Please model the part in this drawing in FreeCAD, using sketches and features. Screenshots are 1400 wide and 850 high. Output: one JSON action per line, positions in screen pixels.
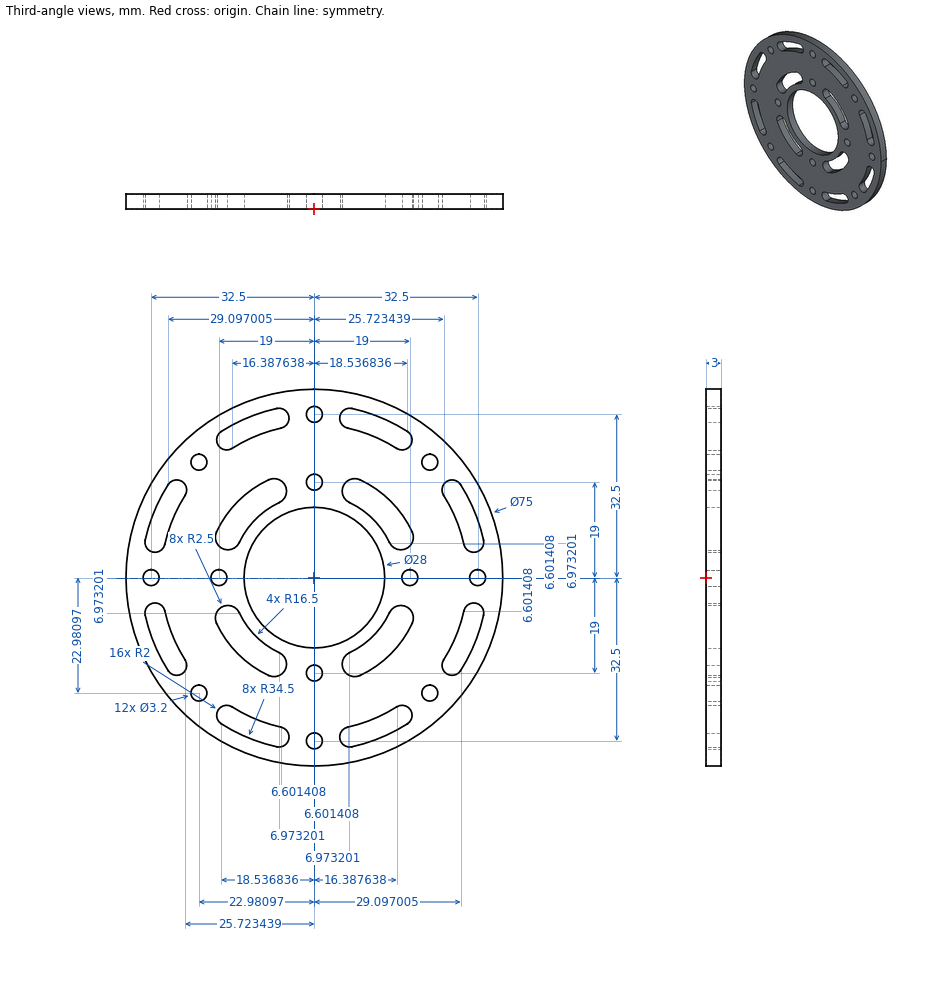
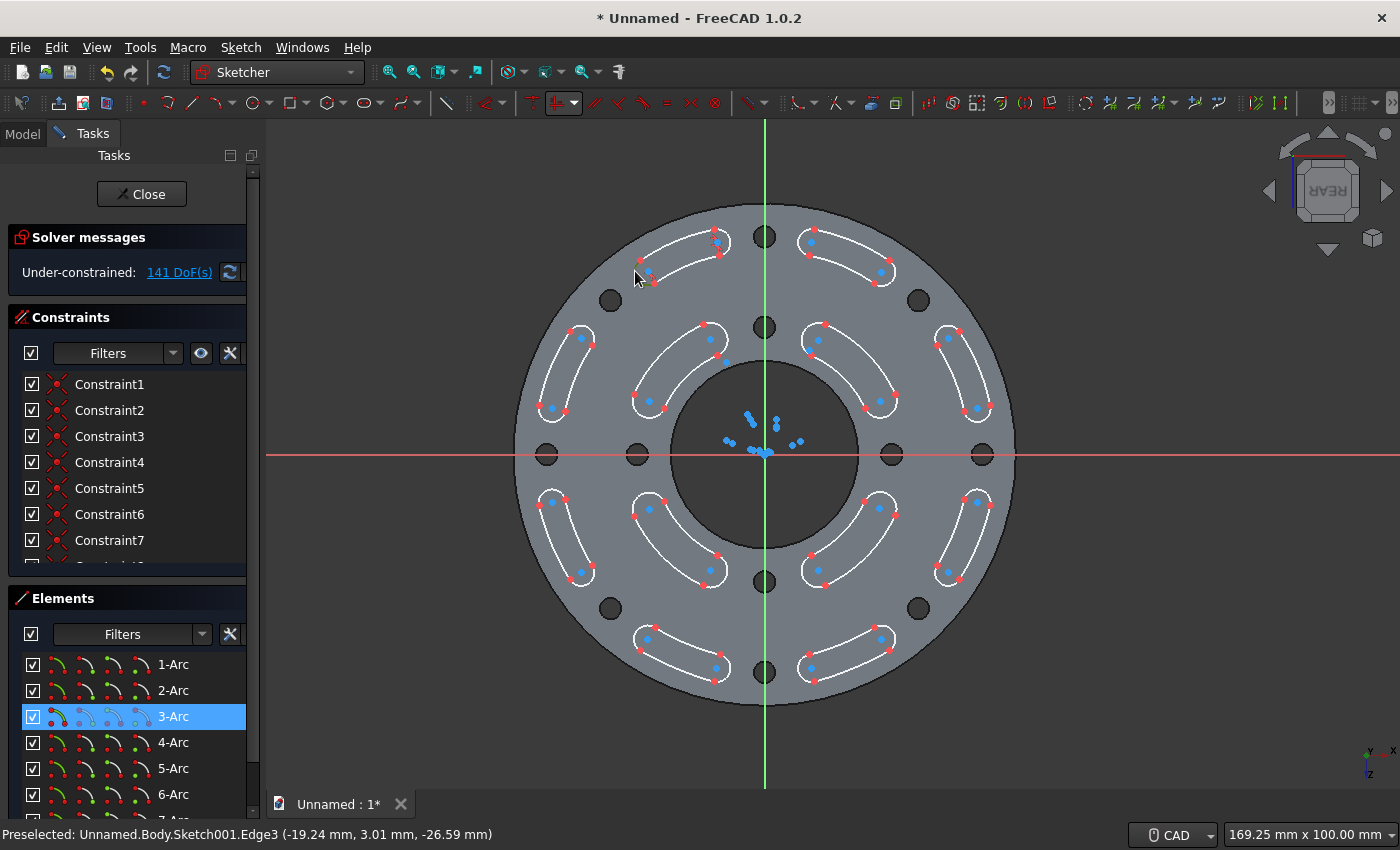
{"action": "left_click", "coordinate": [699, 261]}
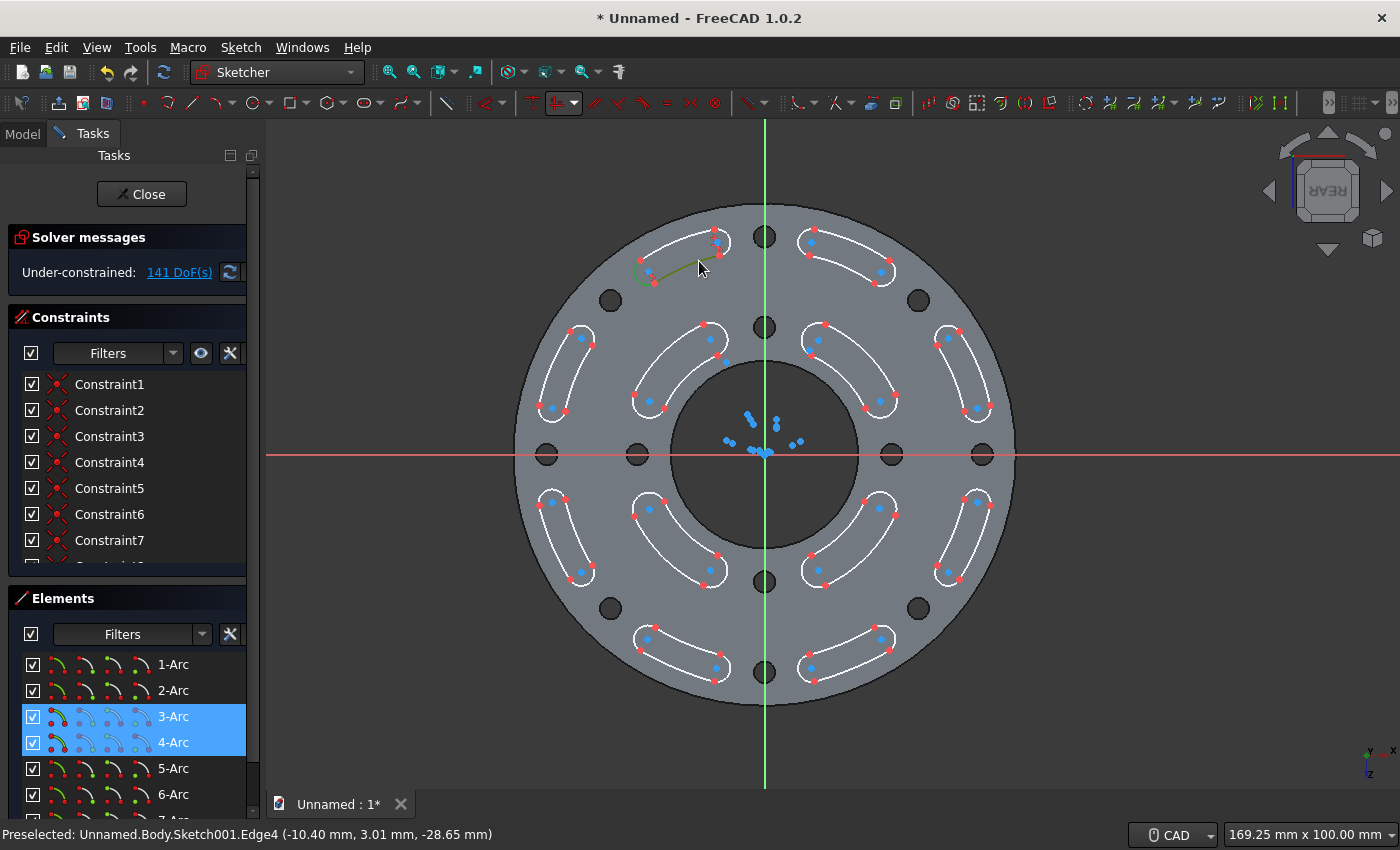
{"action": "left_click", "coordinate": [644, 104]}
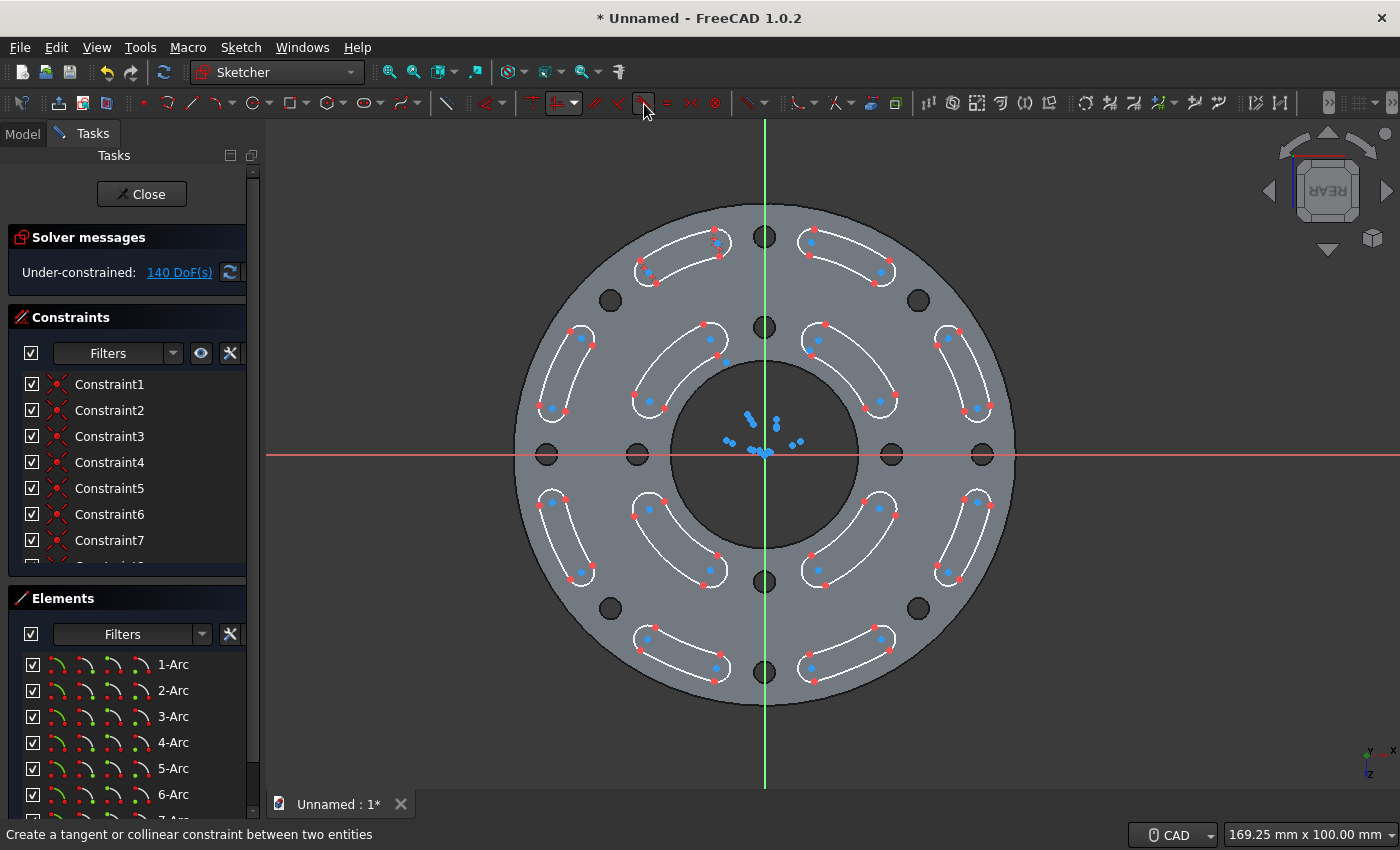
{"action": "left_click", "coordinate": [698, 367]}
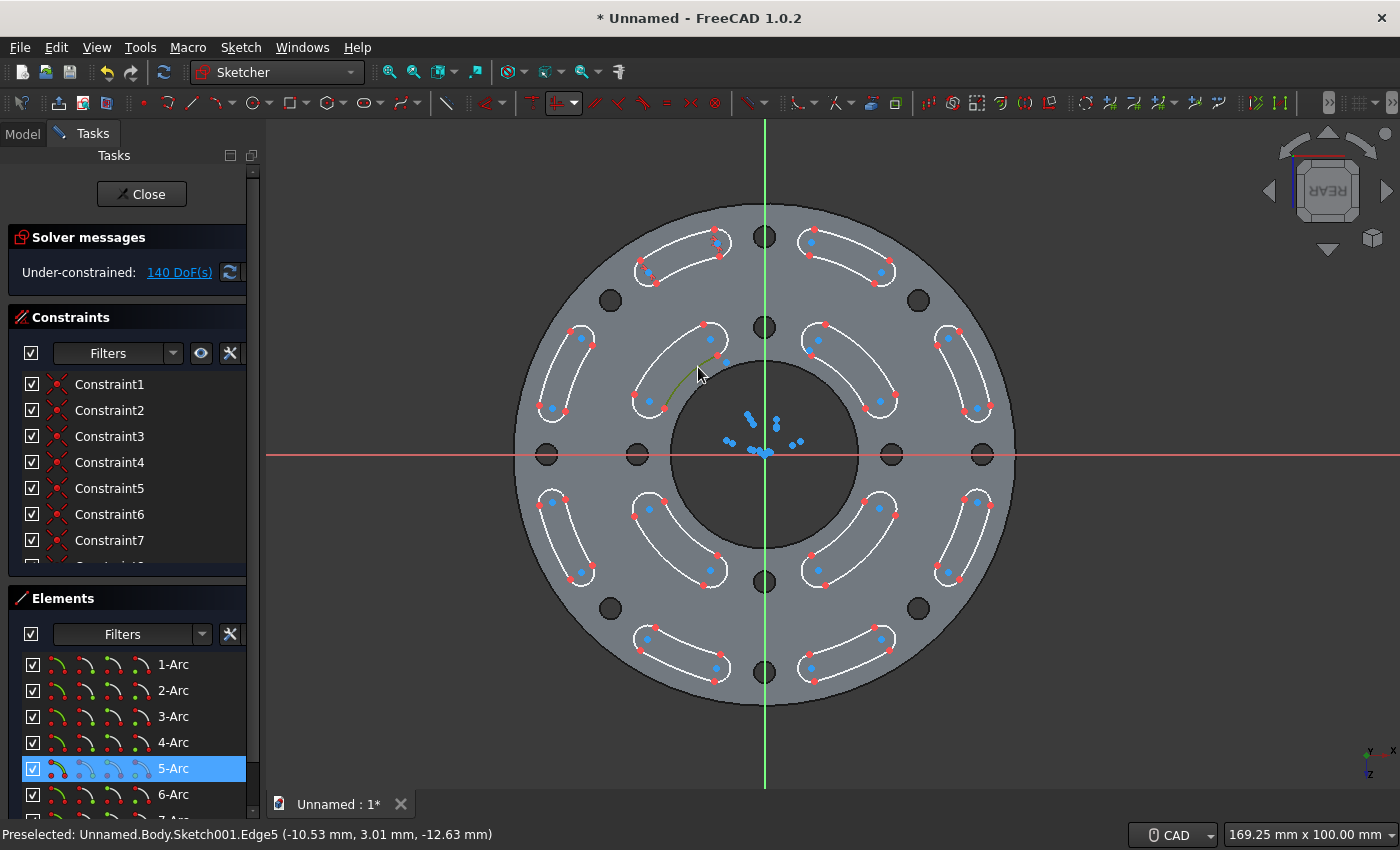
{"action": "left_click", "coordinate": [727, 344]}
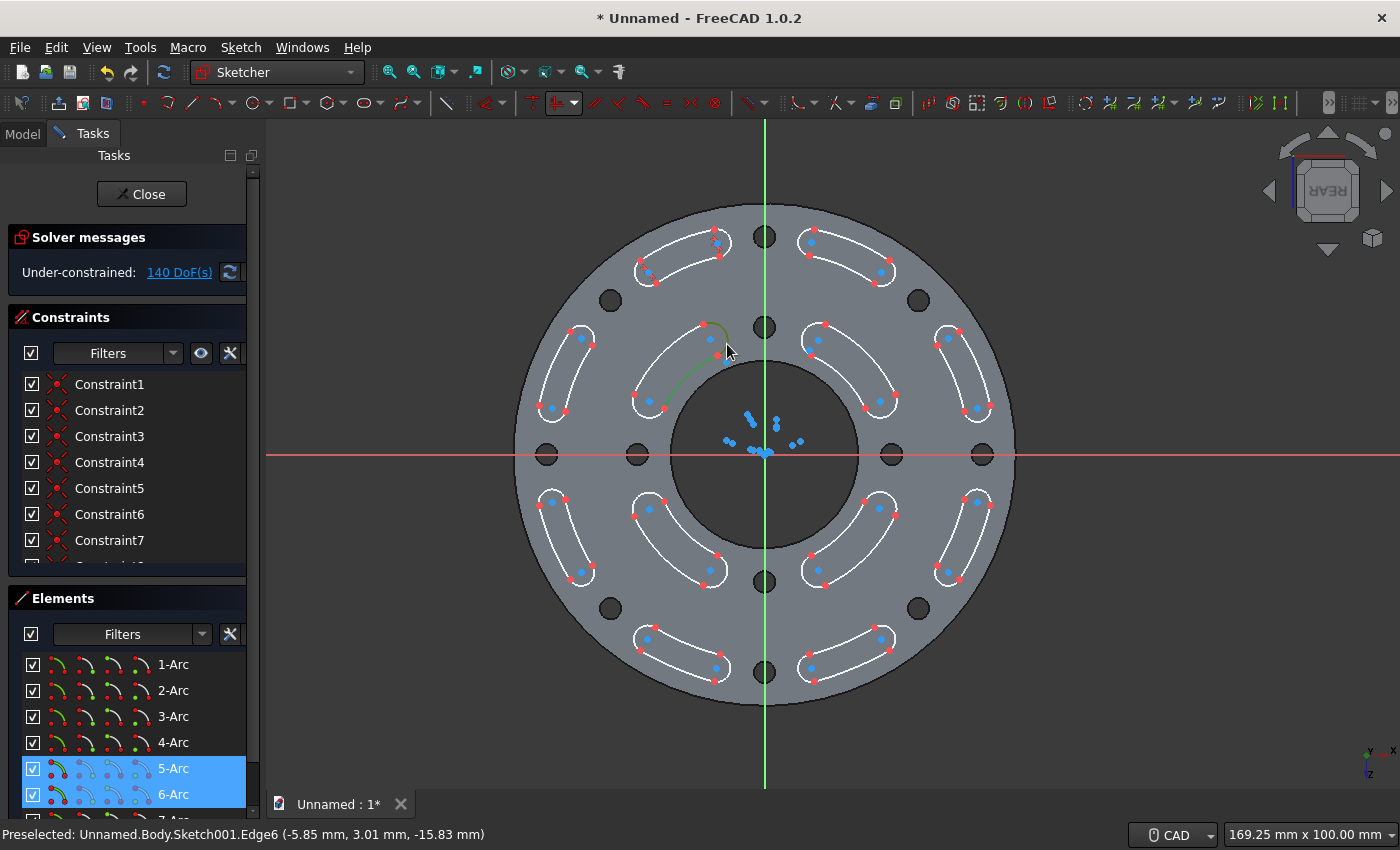
{"action": "left_click", "coordinate": [644, 104]}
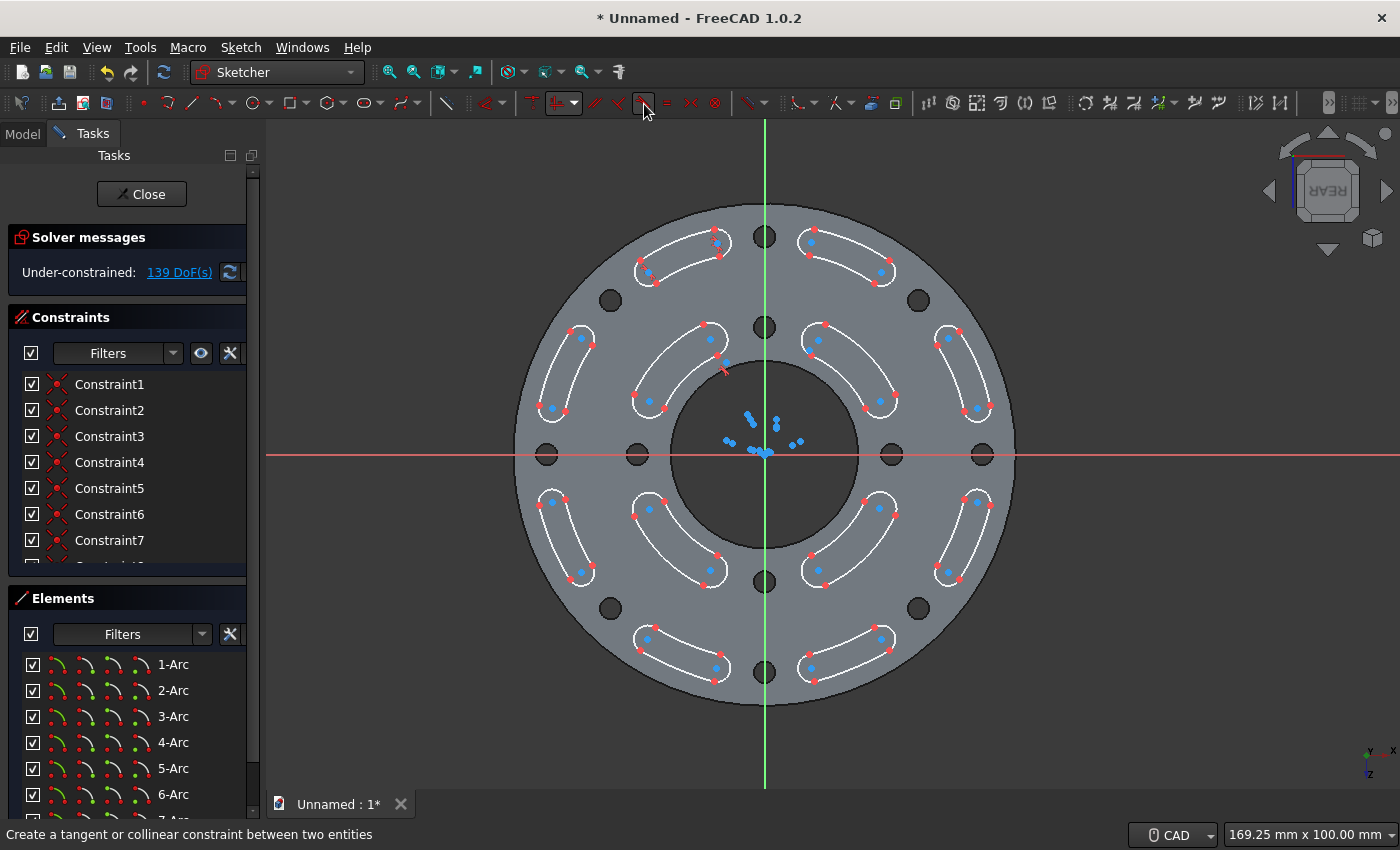
{"action": "left_click", "coordinate": [698, 367]}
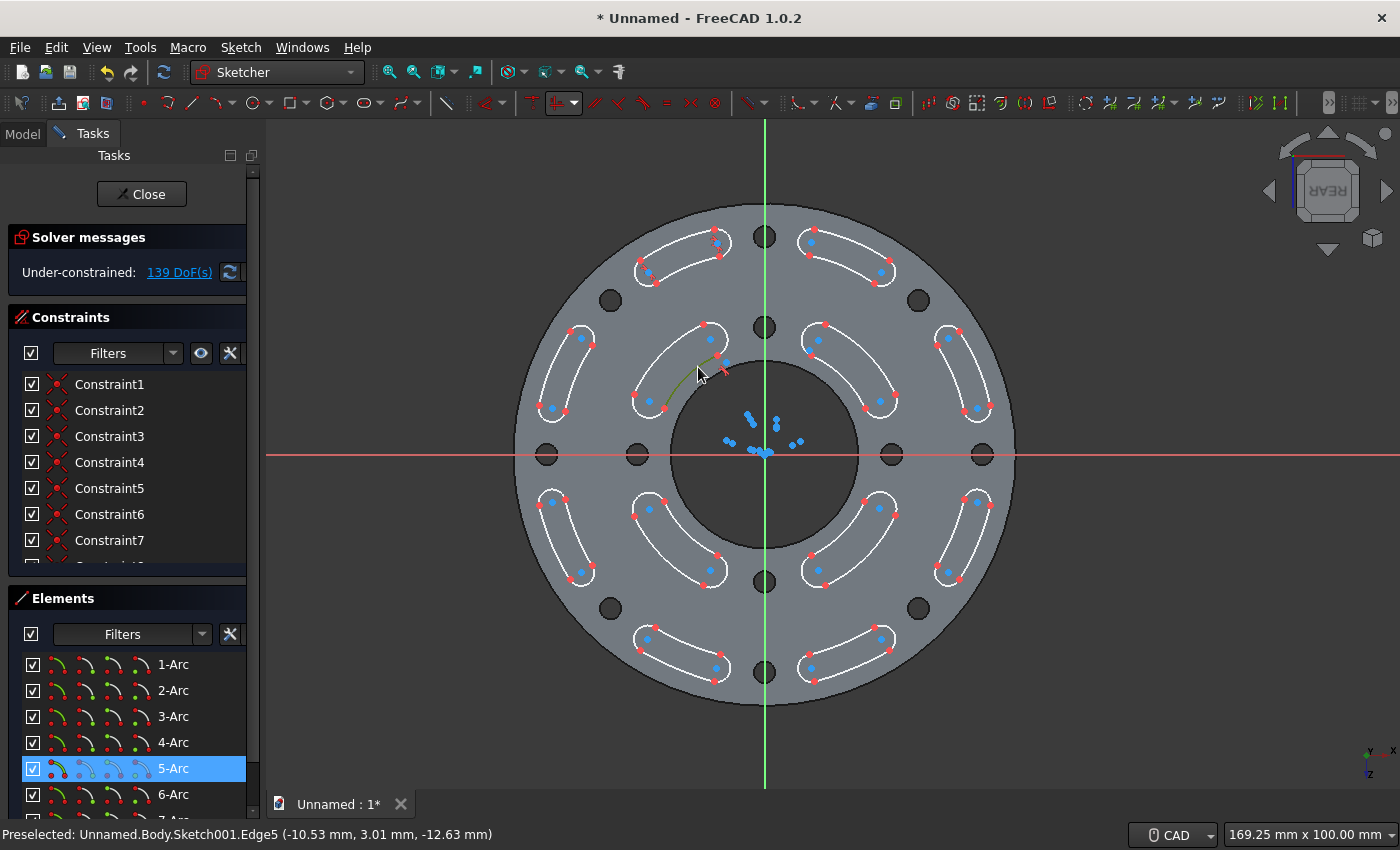
{"action": "left_click", "coordinate": [635, 409]}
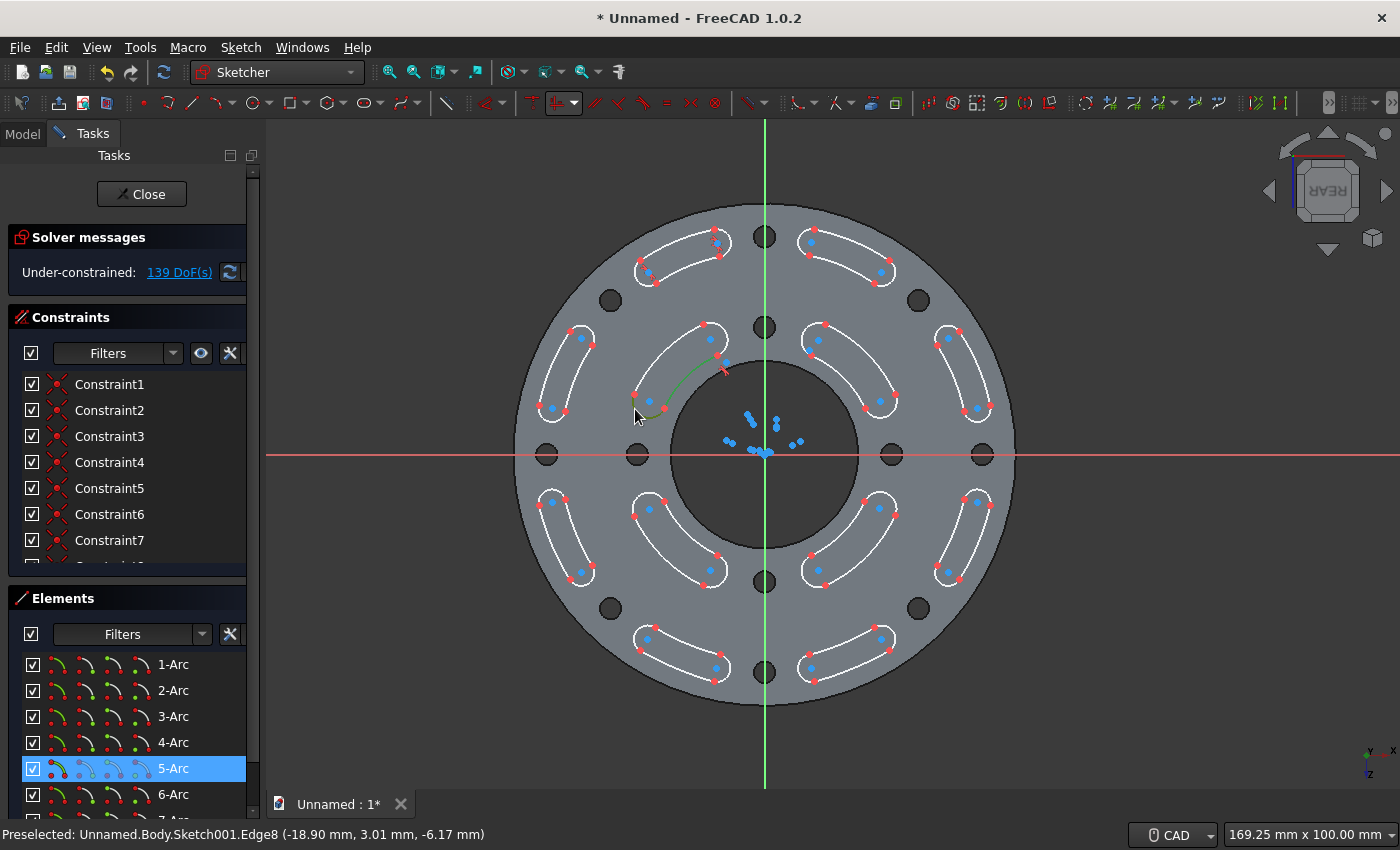
{"action": "left_click", "coordinate": [644, 104]}